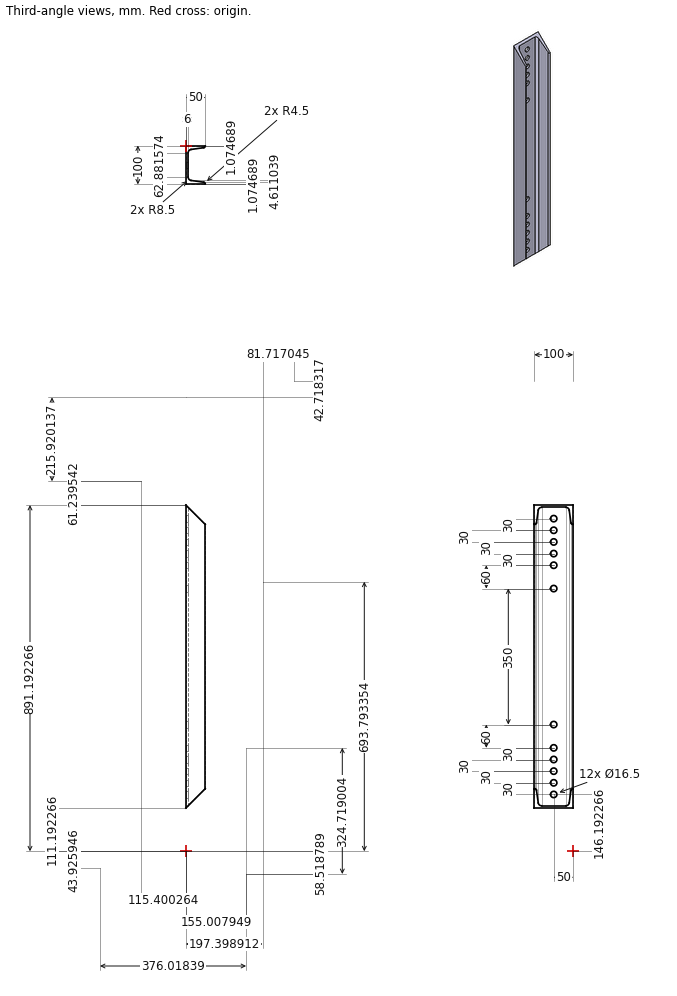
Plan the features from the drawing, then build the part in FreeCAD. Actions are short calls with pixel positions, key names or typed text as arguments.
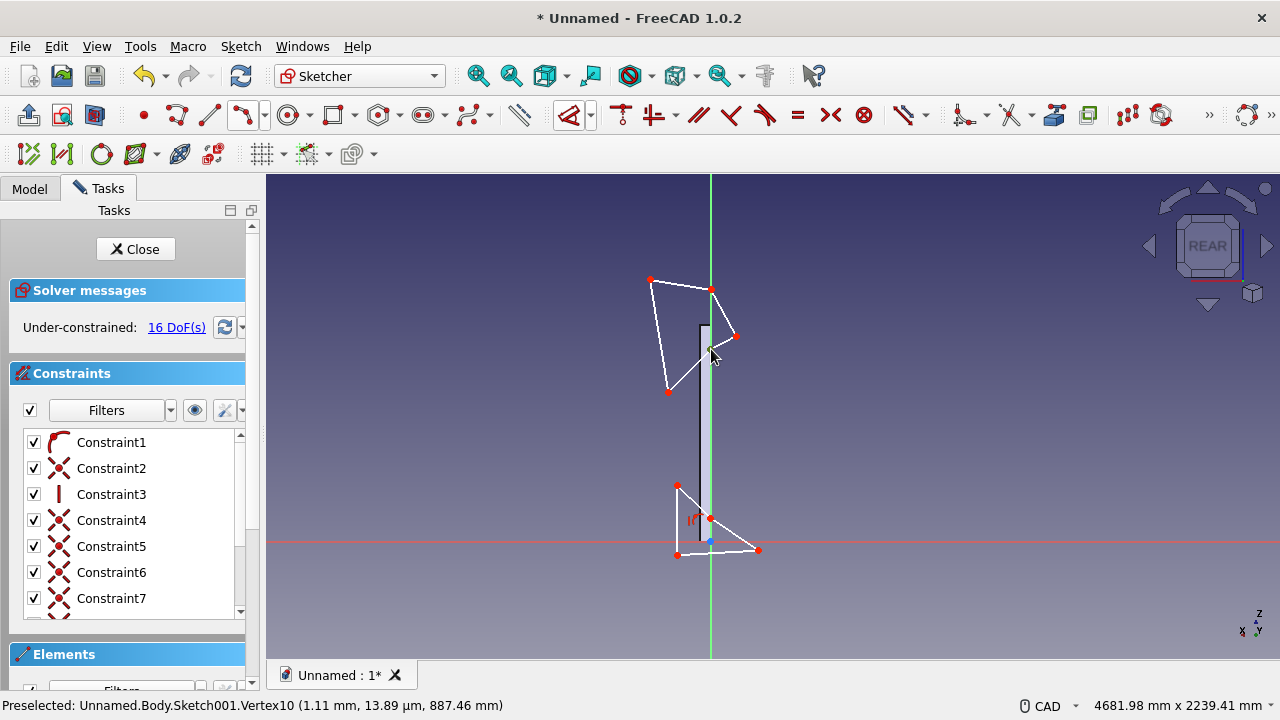
click(711, 600)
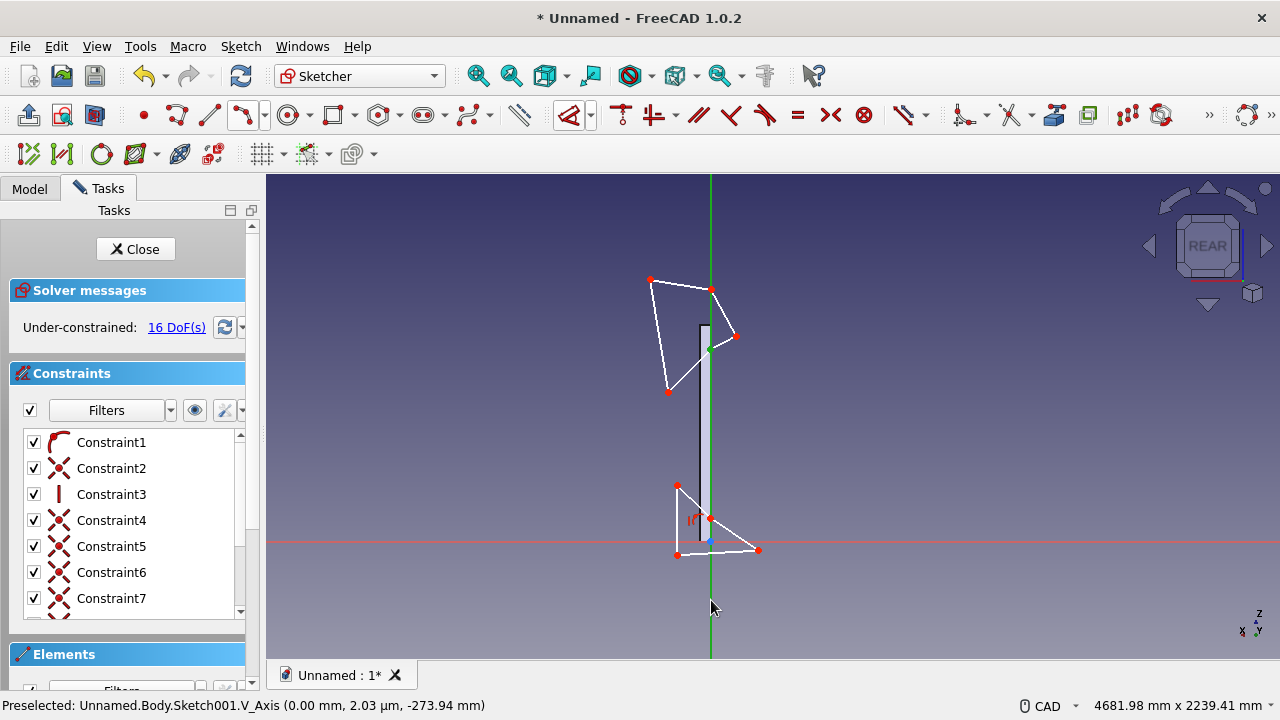
click(621, 116)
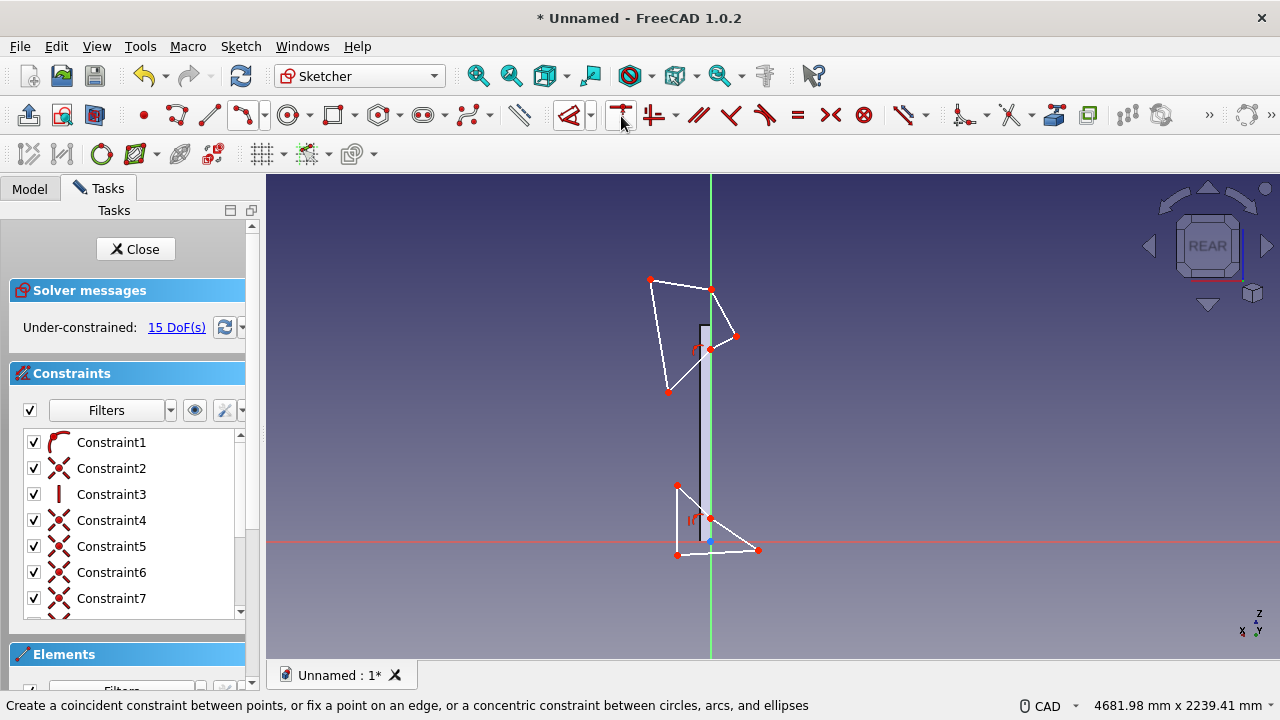
click(711, 290)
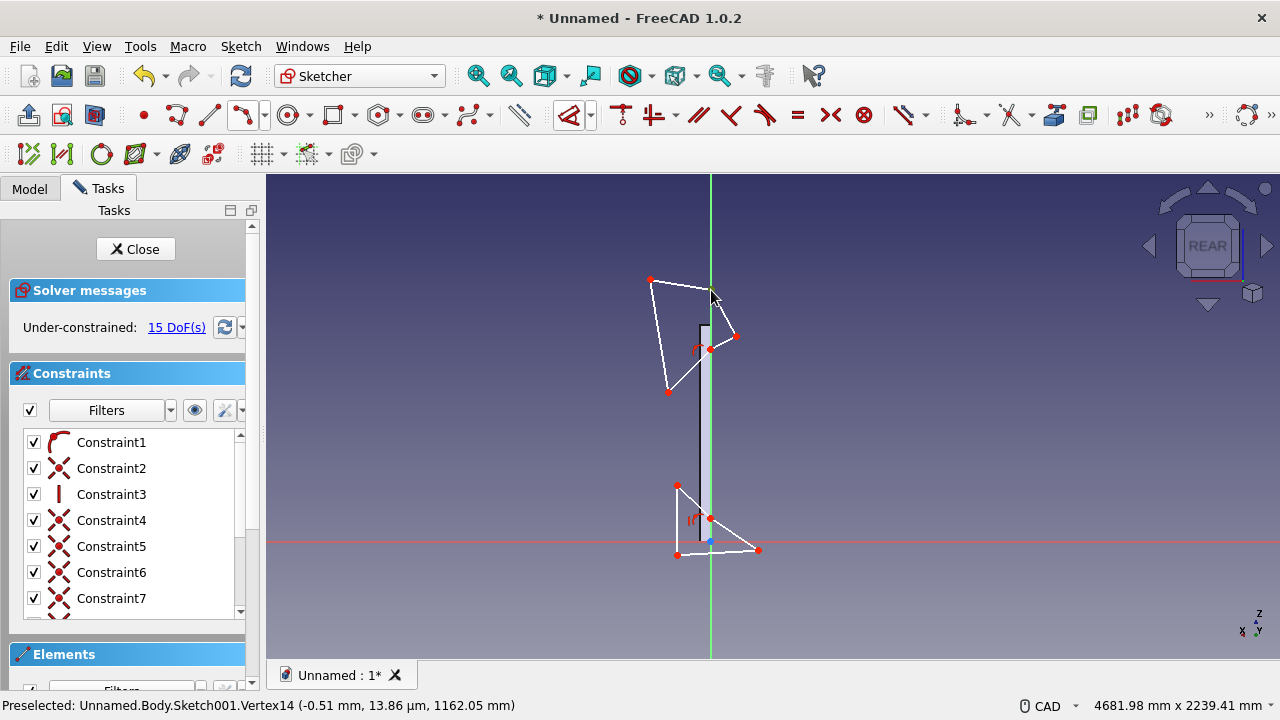
click(711, 600)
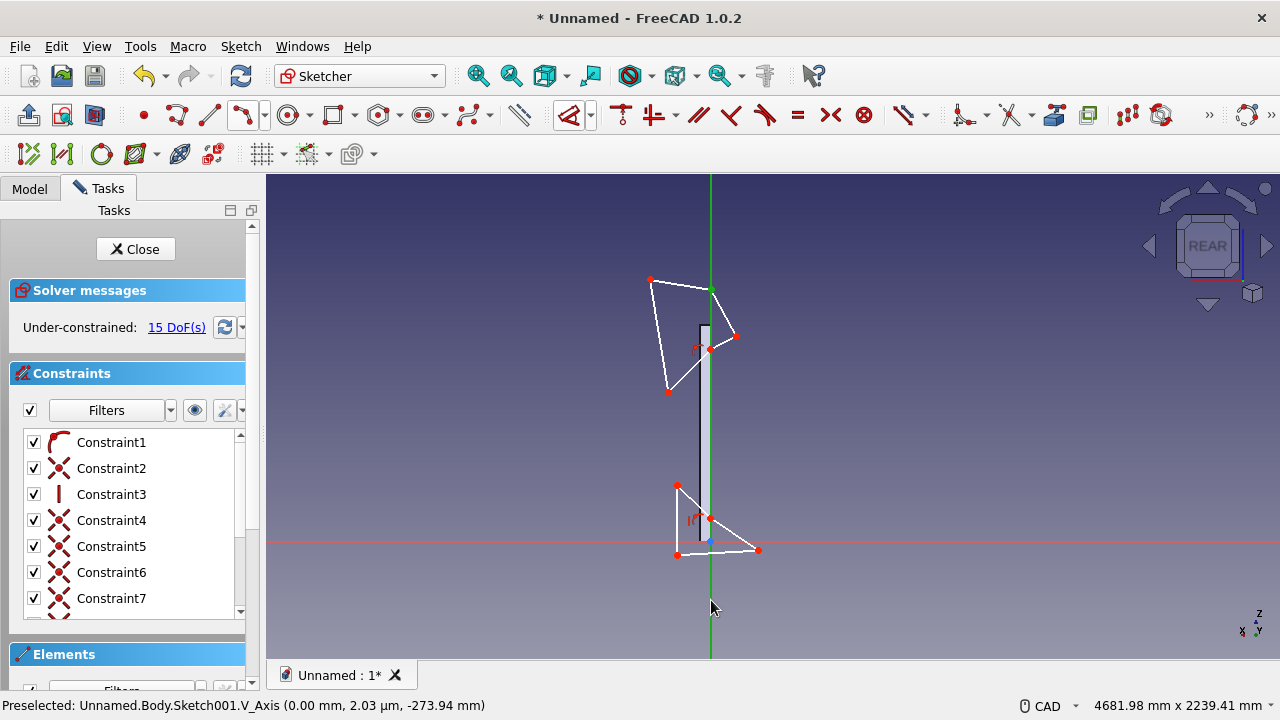
click(621, 116)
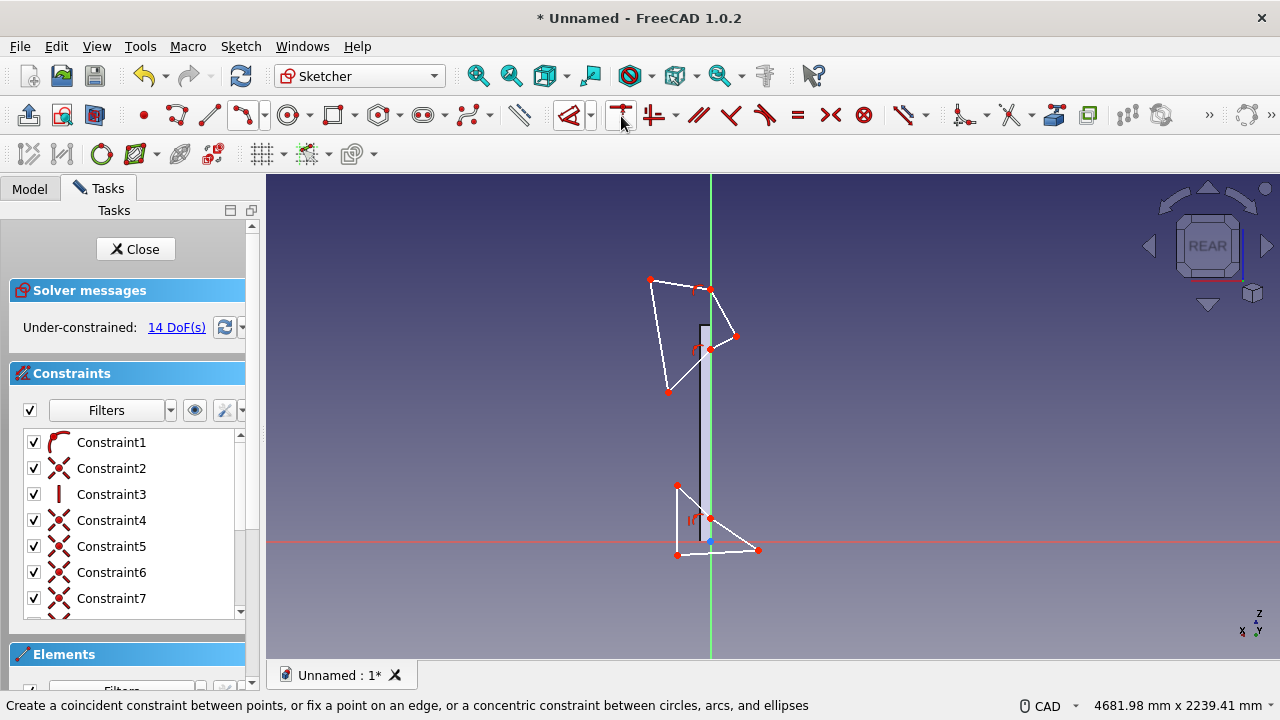
click(677, 506)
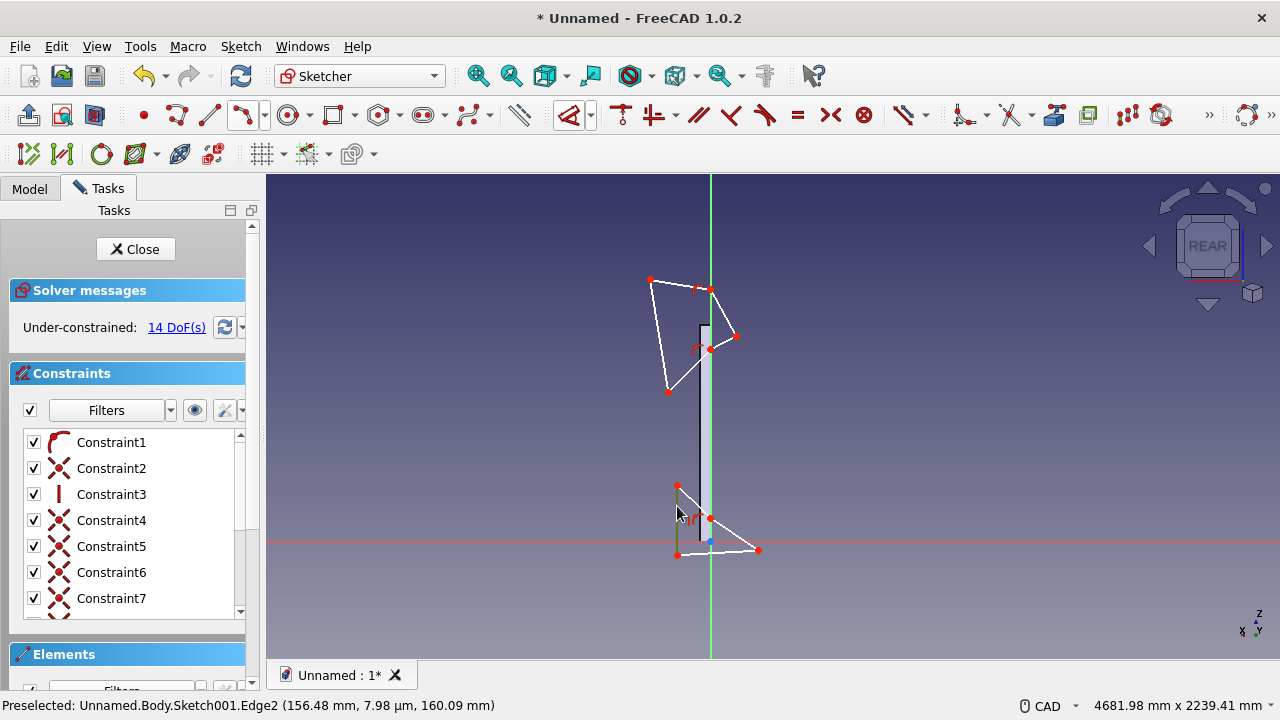
click(590, 116)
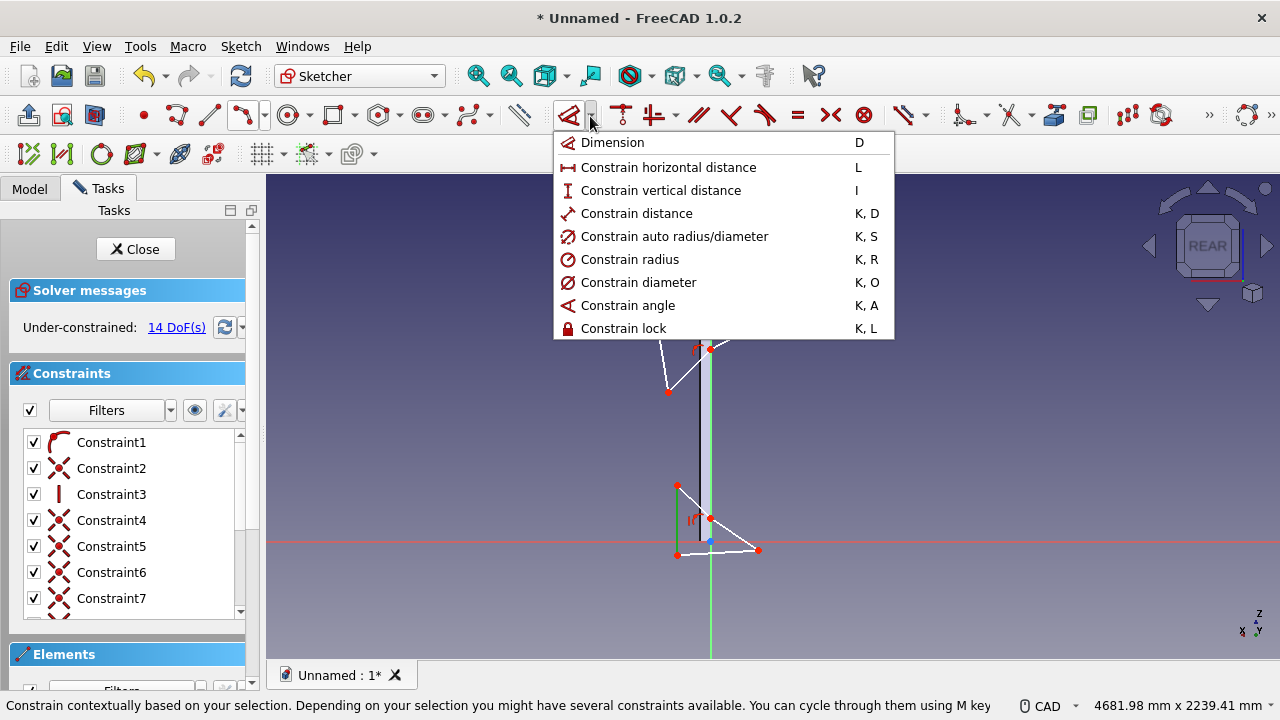
click(724, 190)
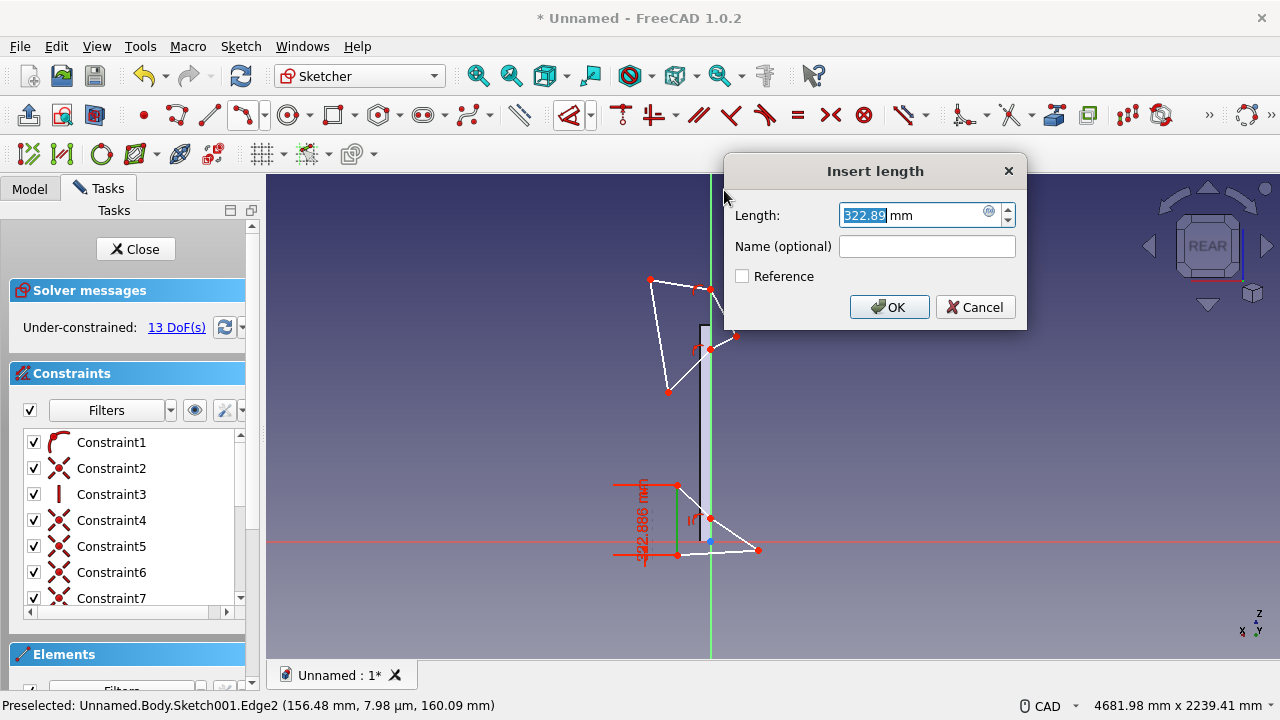
text(324.719004)
key(Return)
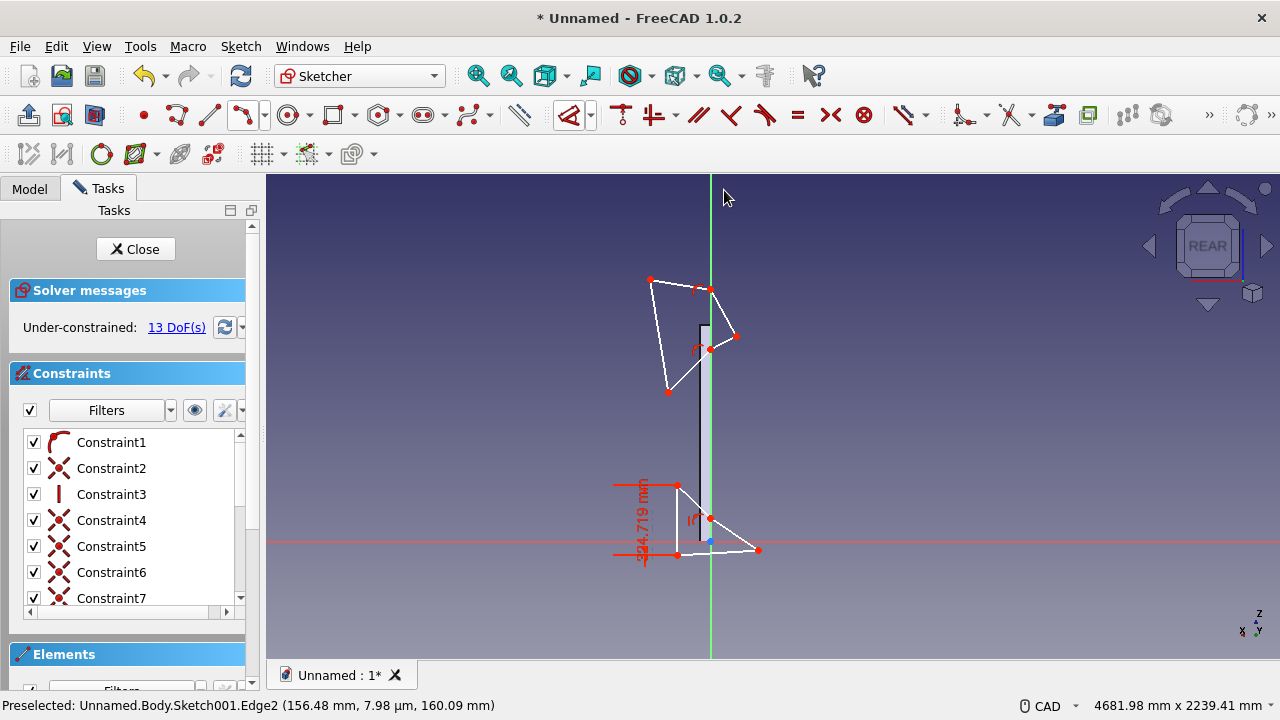
scroll(677, 555, up, 6)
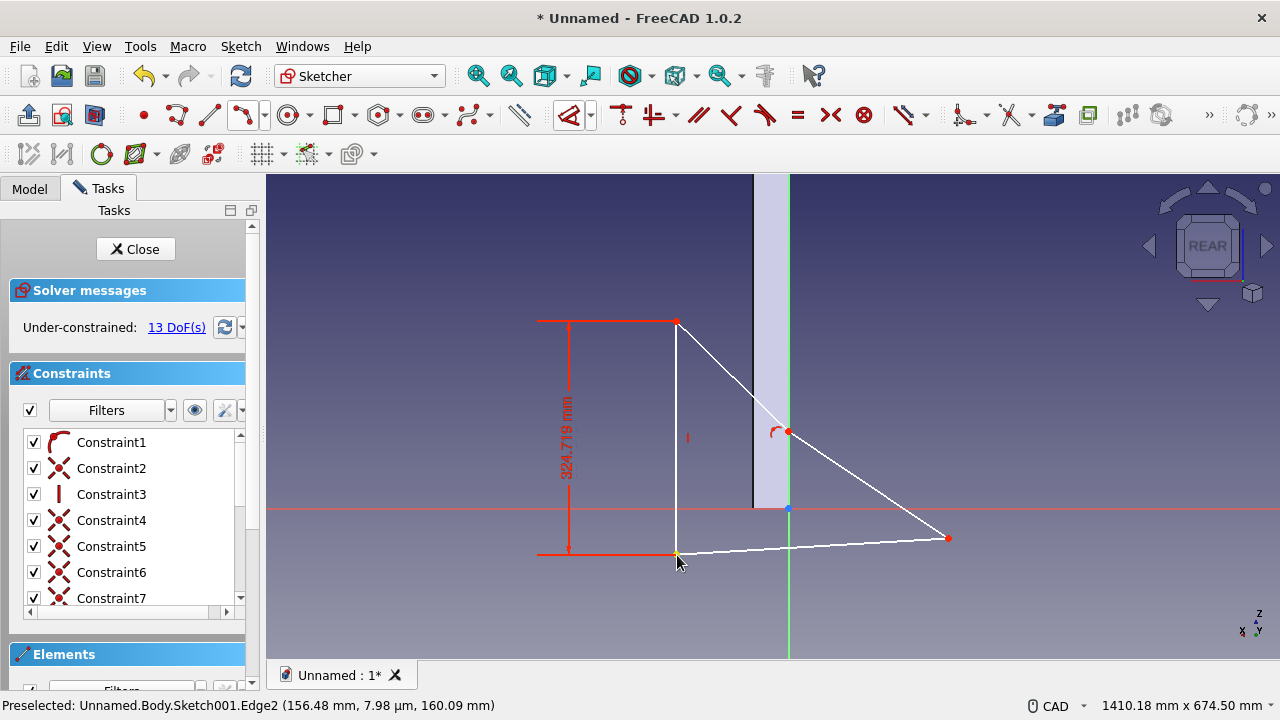
click(676, 555)